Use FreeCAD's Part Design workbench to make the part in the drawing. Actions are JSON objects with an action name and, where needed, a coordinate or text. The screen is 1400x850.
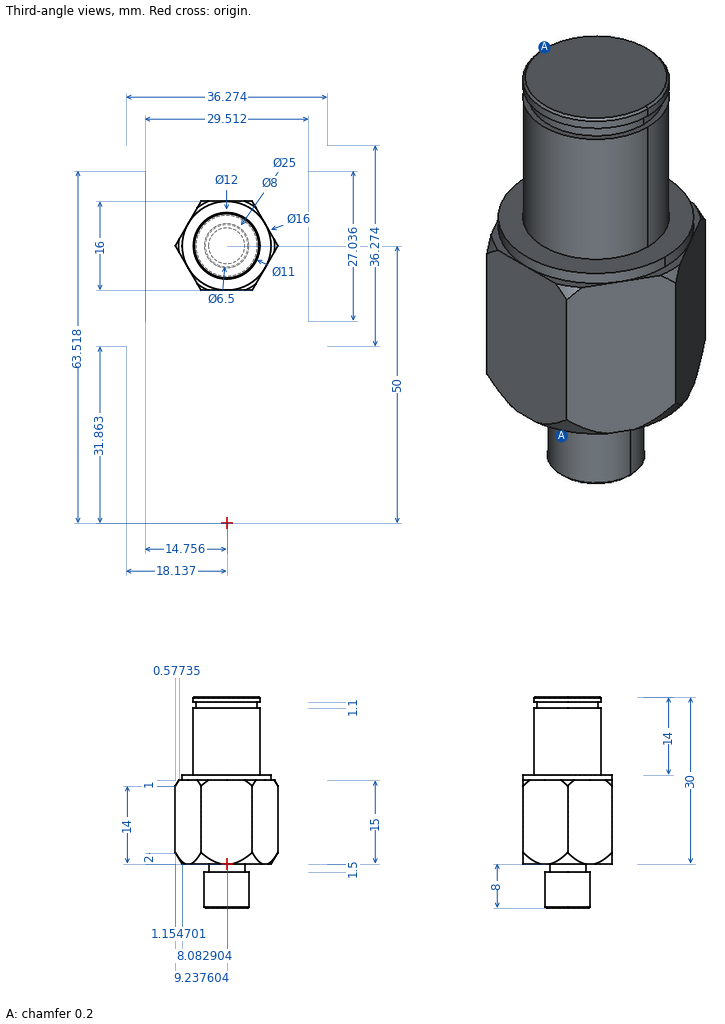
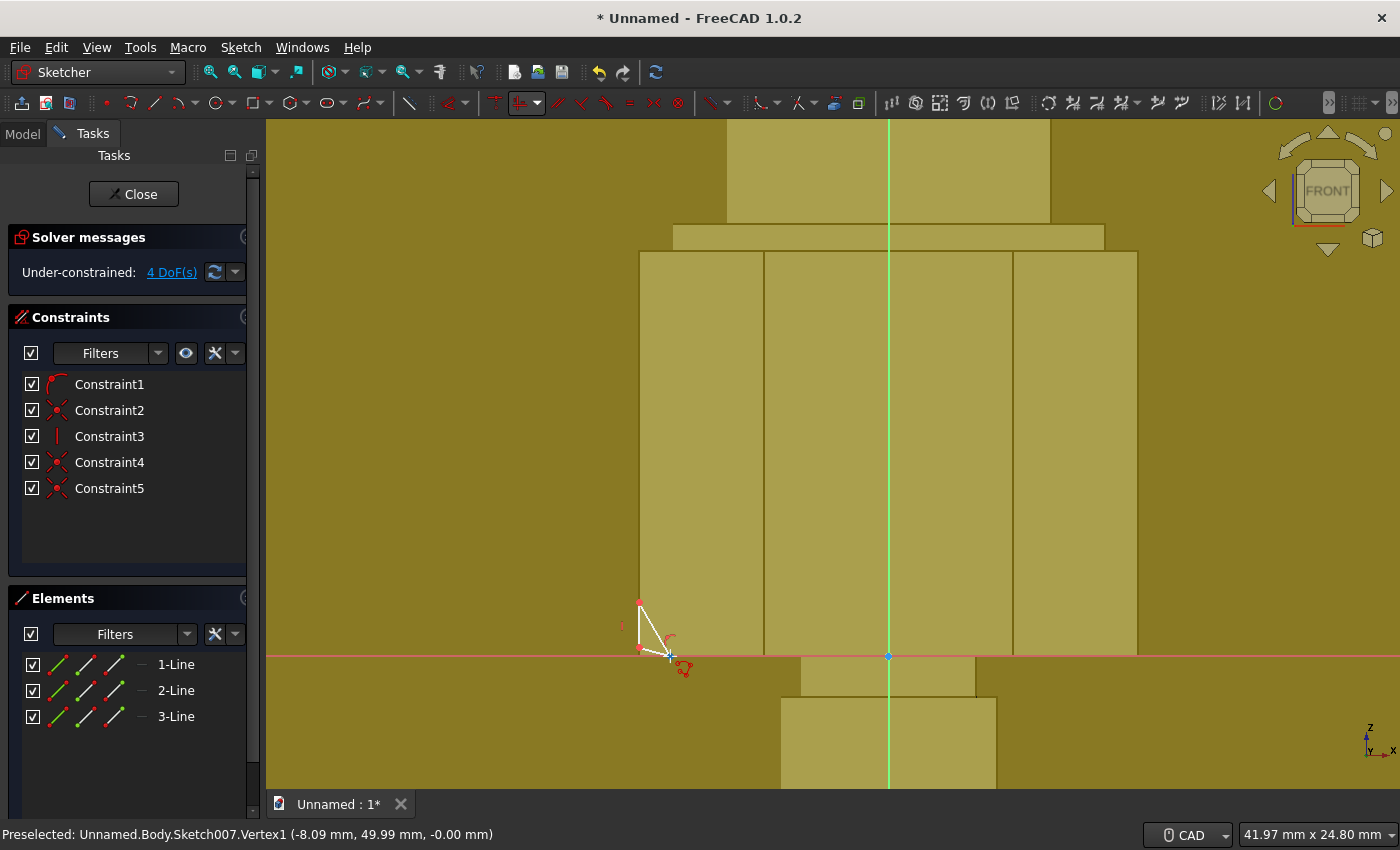
{"action": "left_click", "coordinate": [639, 278]}
{"action": "left_click", "coordinate": [639, 251]}
{"action": "left_click", "coordinate": [655, 251]}
{"action": "left_click", "coordinate": [639, 279]}
{"action": "key", "text": "Escape"}
{"action": "key", "text": "Escape"}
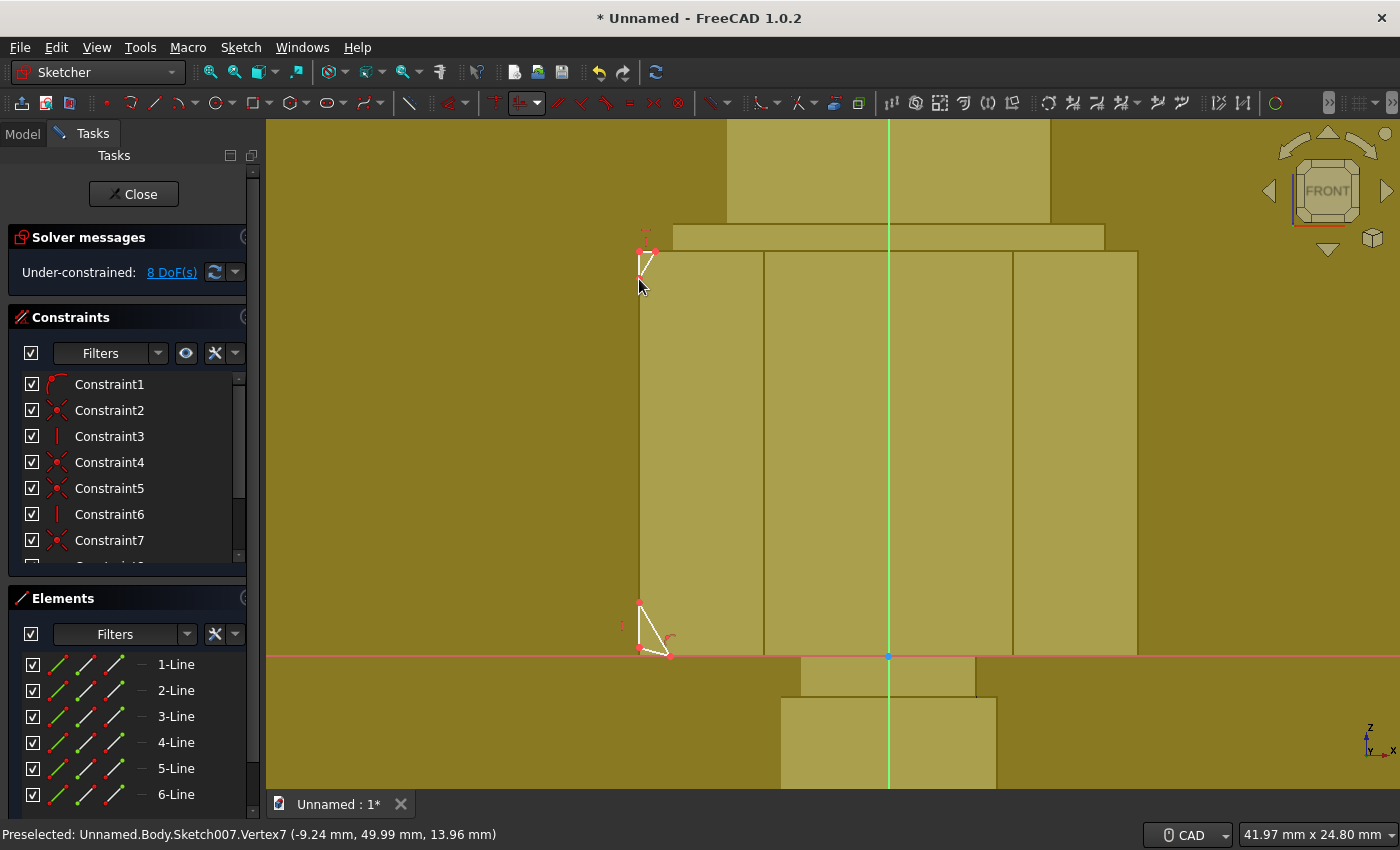
{"action": "scroll", "coordinate": [658, 653], "scroll_direction": "up", "scroll_amount": 3}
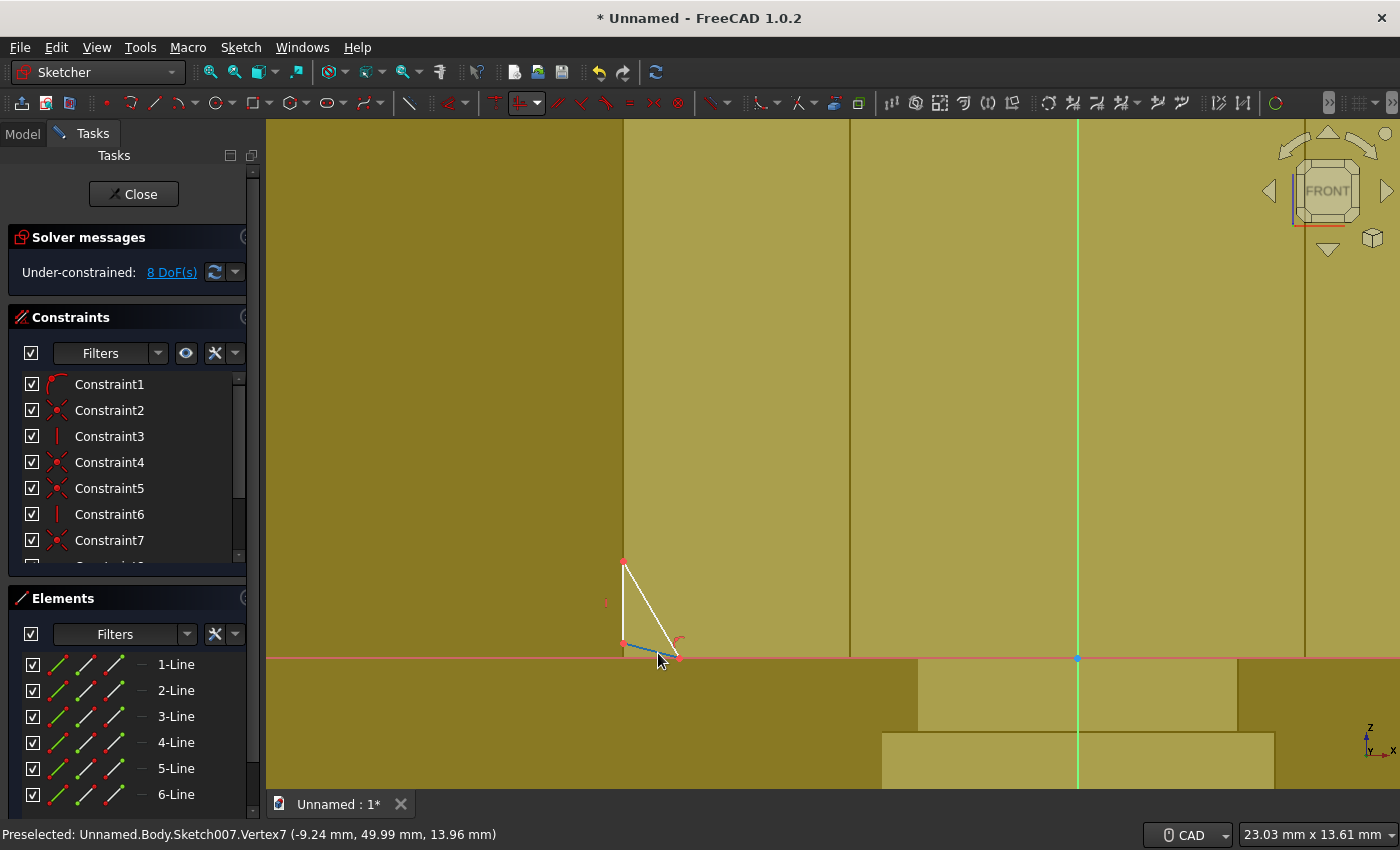
{"action": "left_click", "coordinate": [657, 652]}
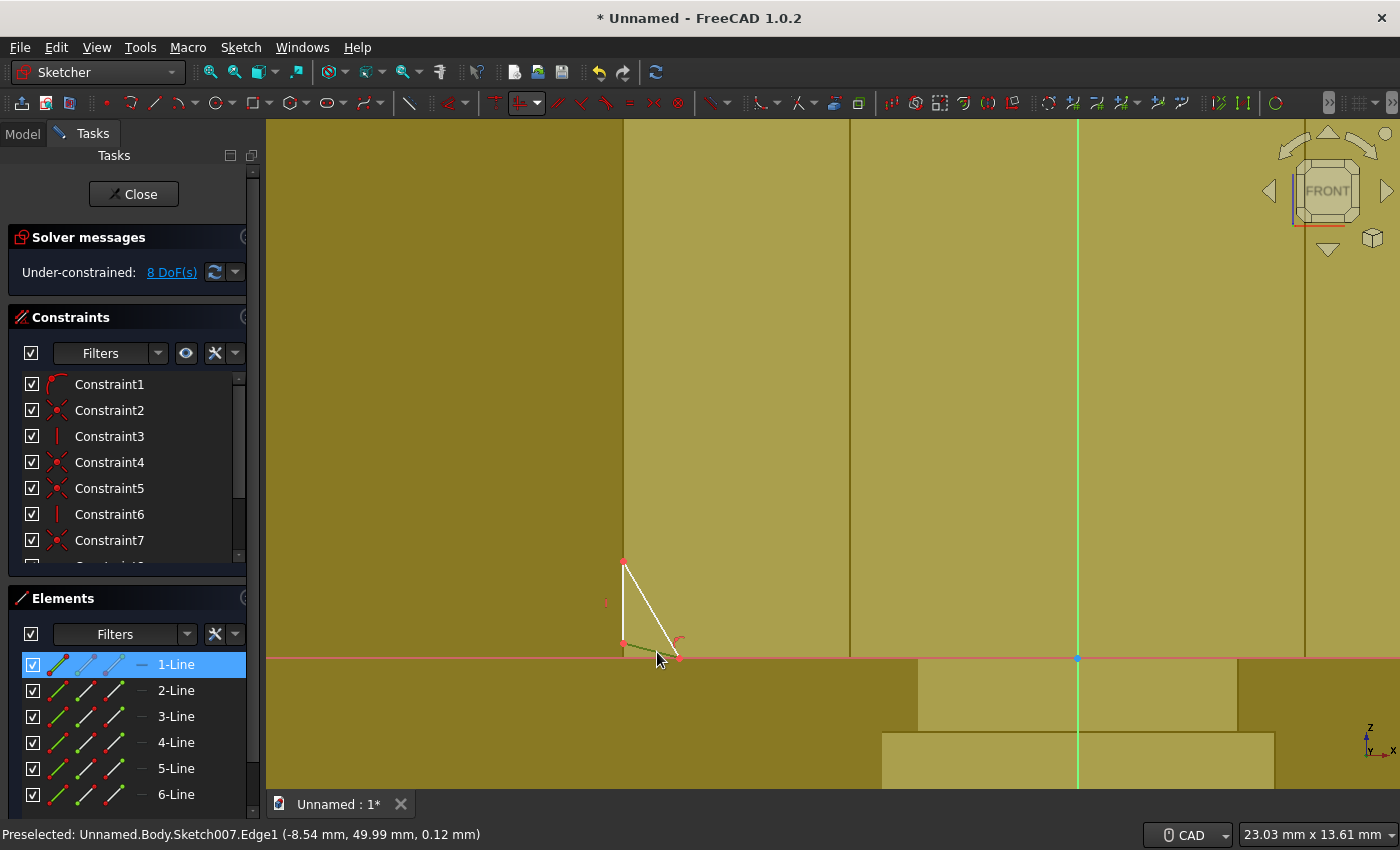
{"action": "left_click", "coordinate": [540, 104]}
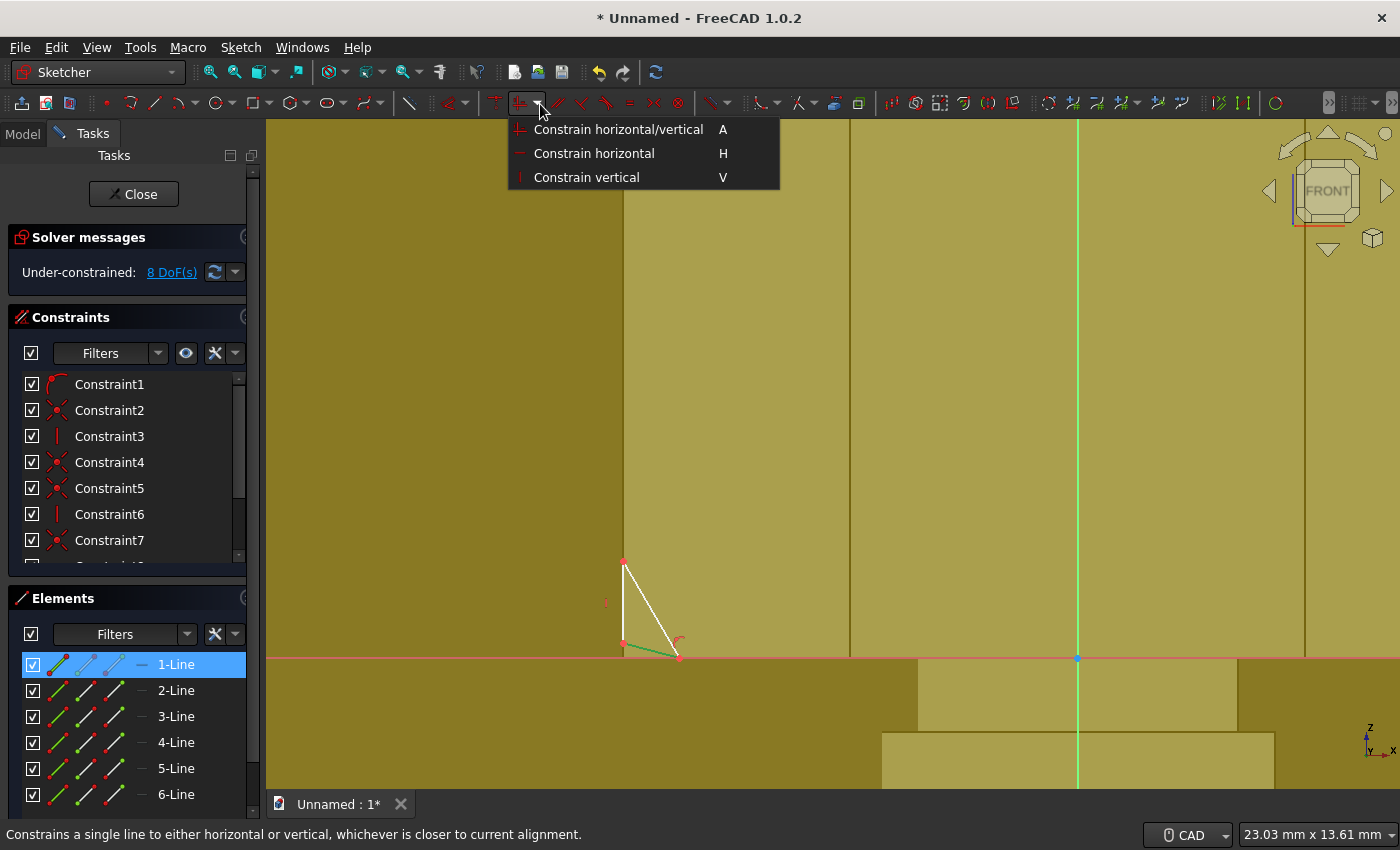
{"action": "left_click", "coordinate": [644, 153]}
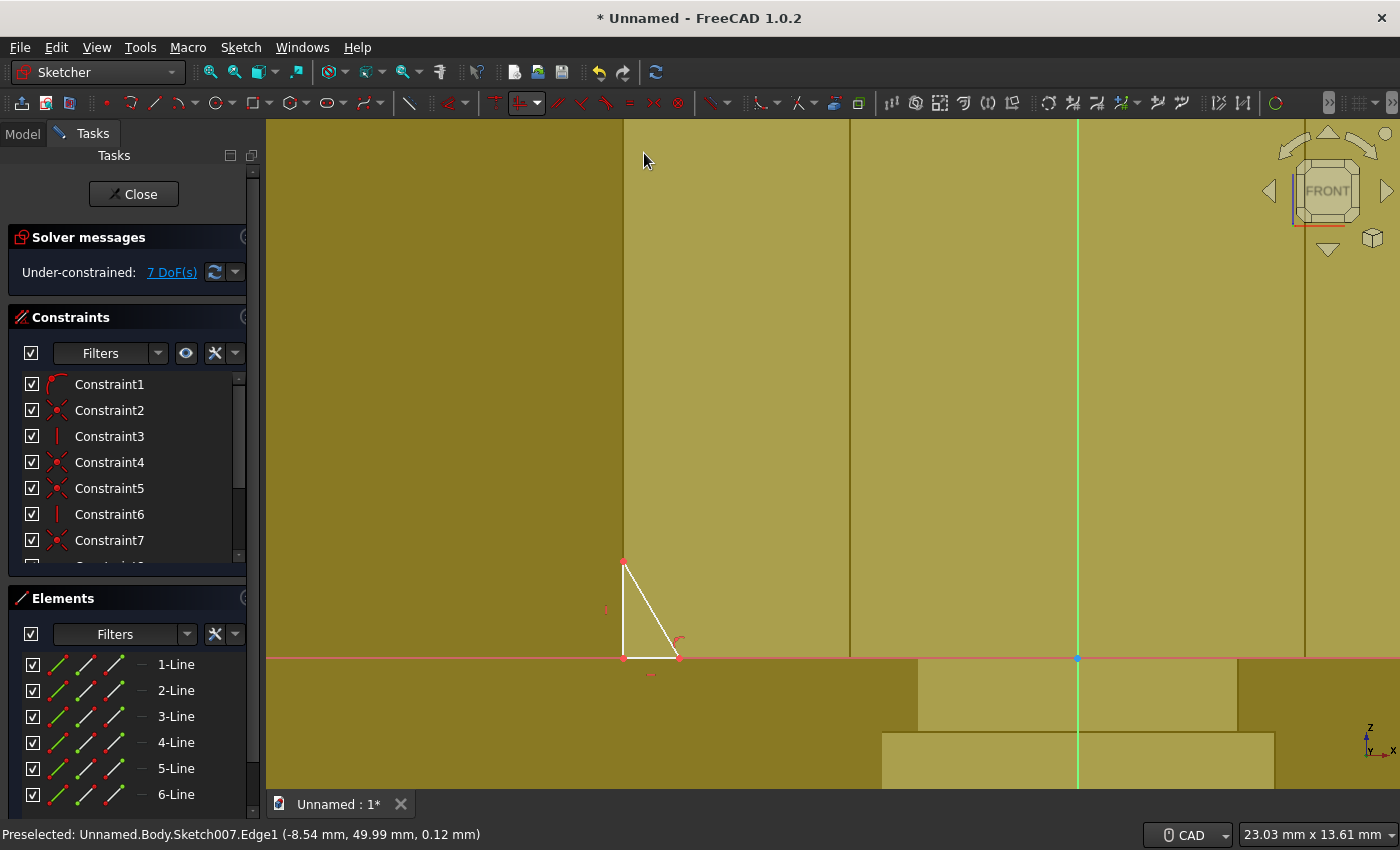
{"action": "left_click", "coordinate": [448, 104]}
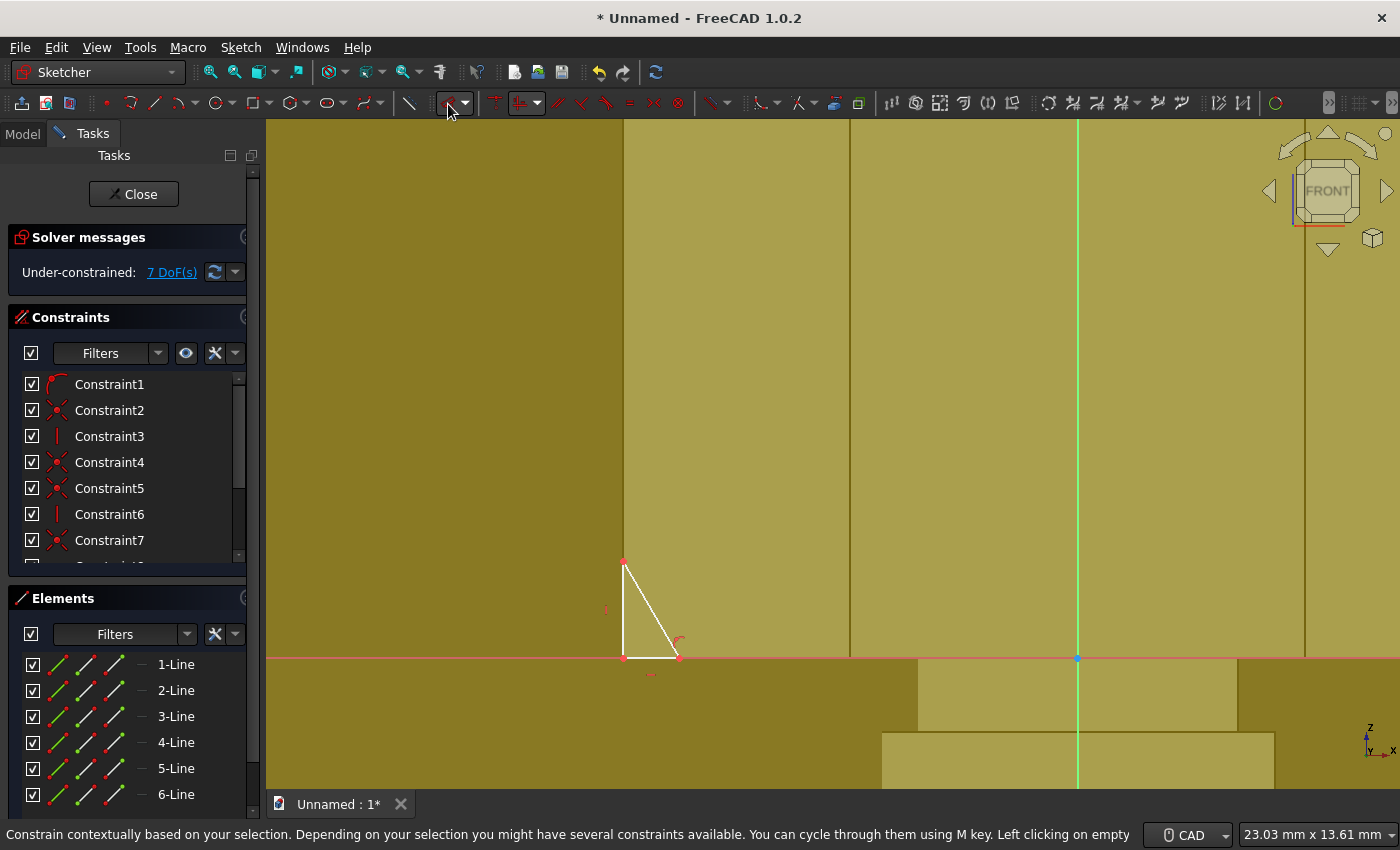
{"action": "left_click", "coordinate": [623, 629]}
{"action": "left_click", "coordinate": [589, 610]}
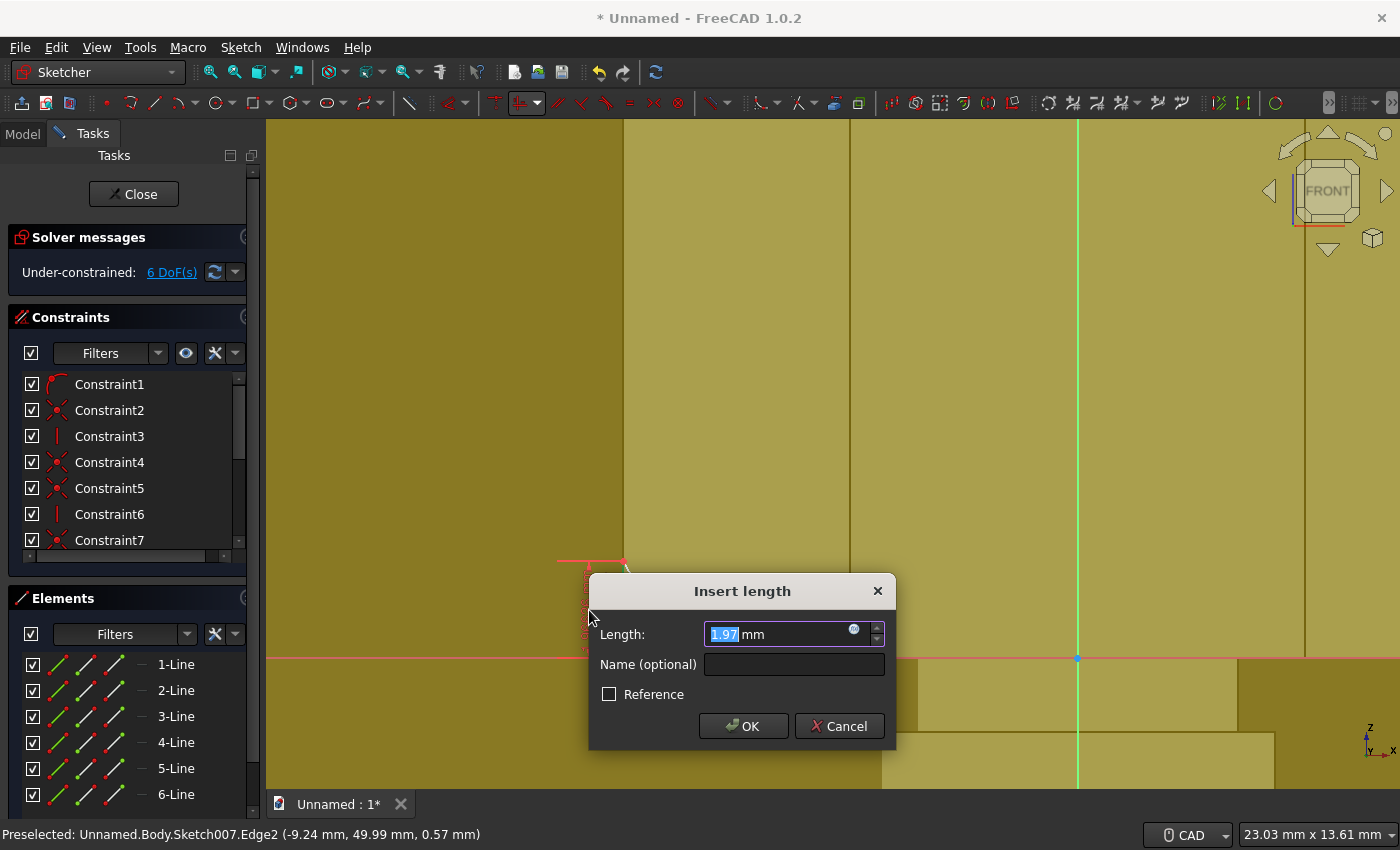
{"action": "type", "text": "2"}
{"action": "key", "text": "Return"}